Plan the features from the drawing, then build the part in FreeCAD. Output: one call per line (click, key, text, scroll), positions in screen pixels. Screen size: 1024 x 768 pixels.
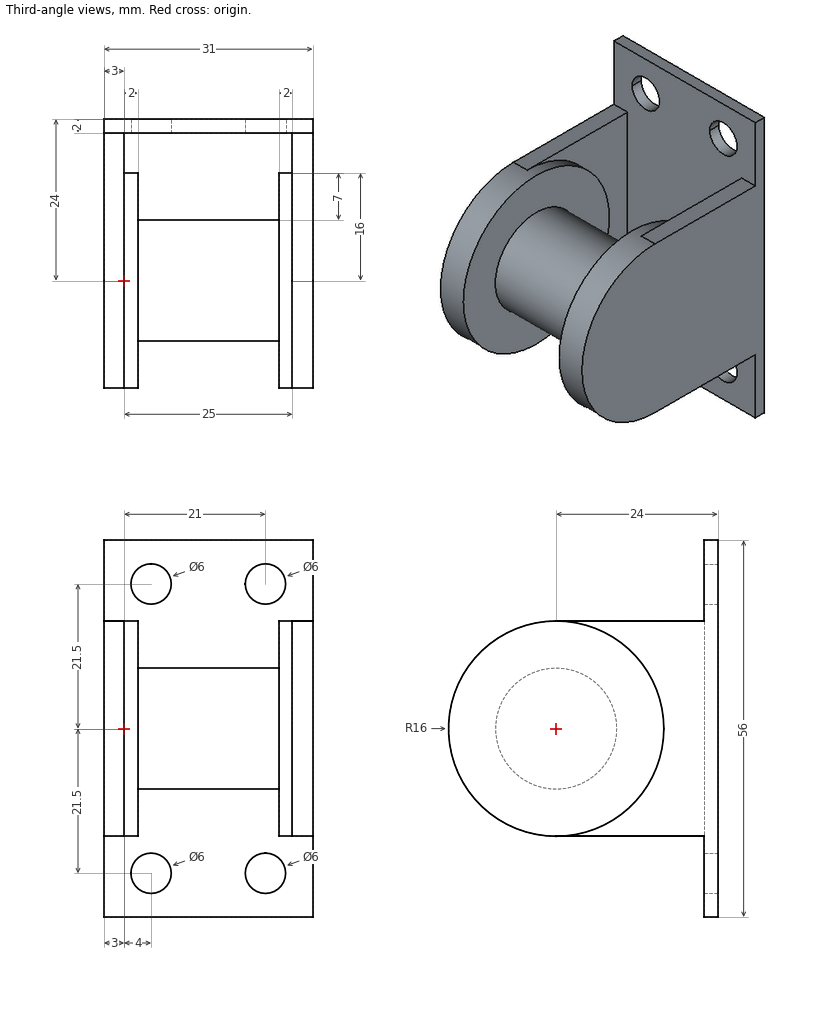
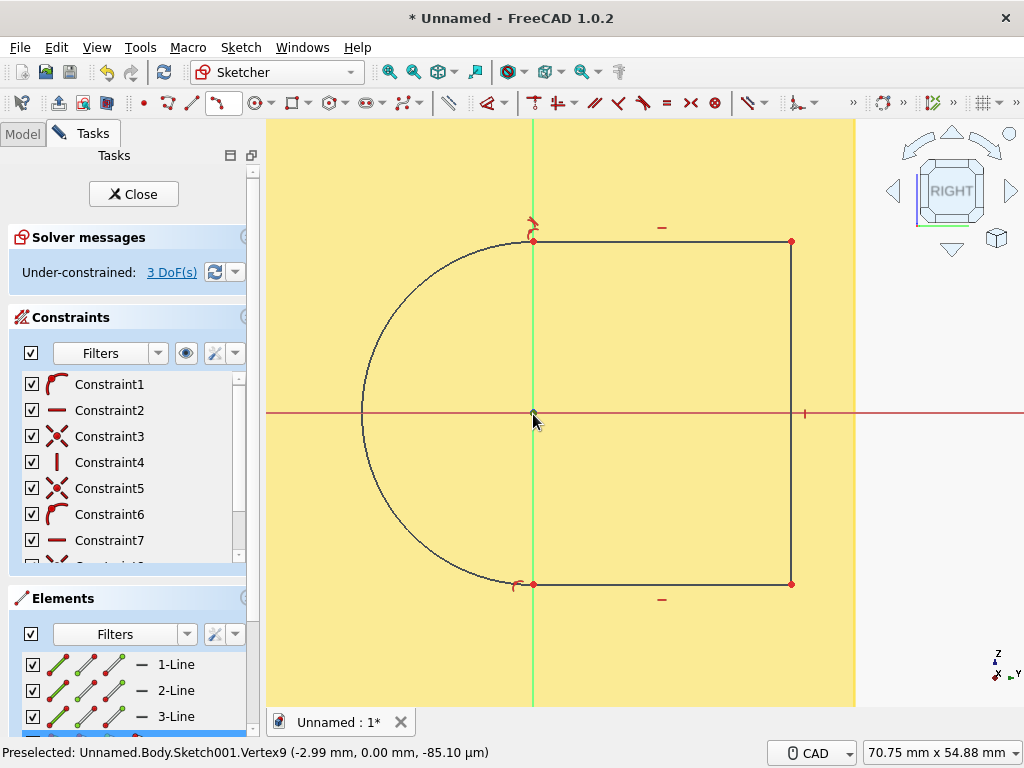
click(415, 413)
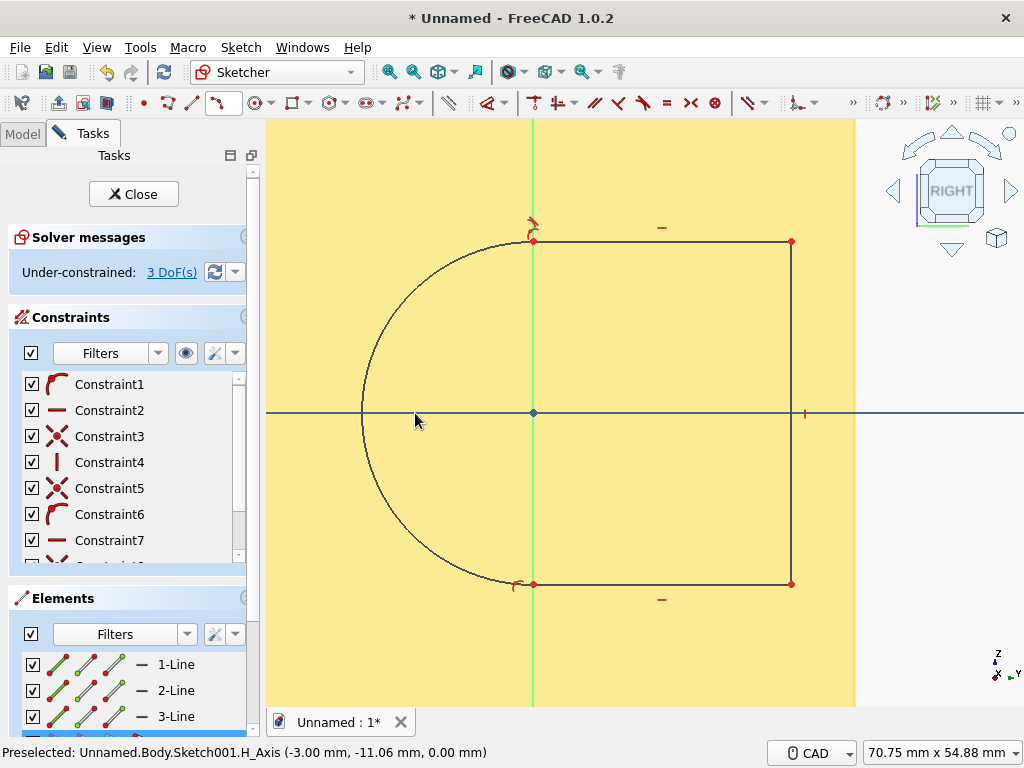
click(534, 104)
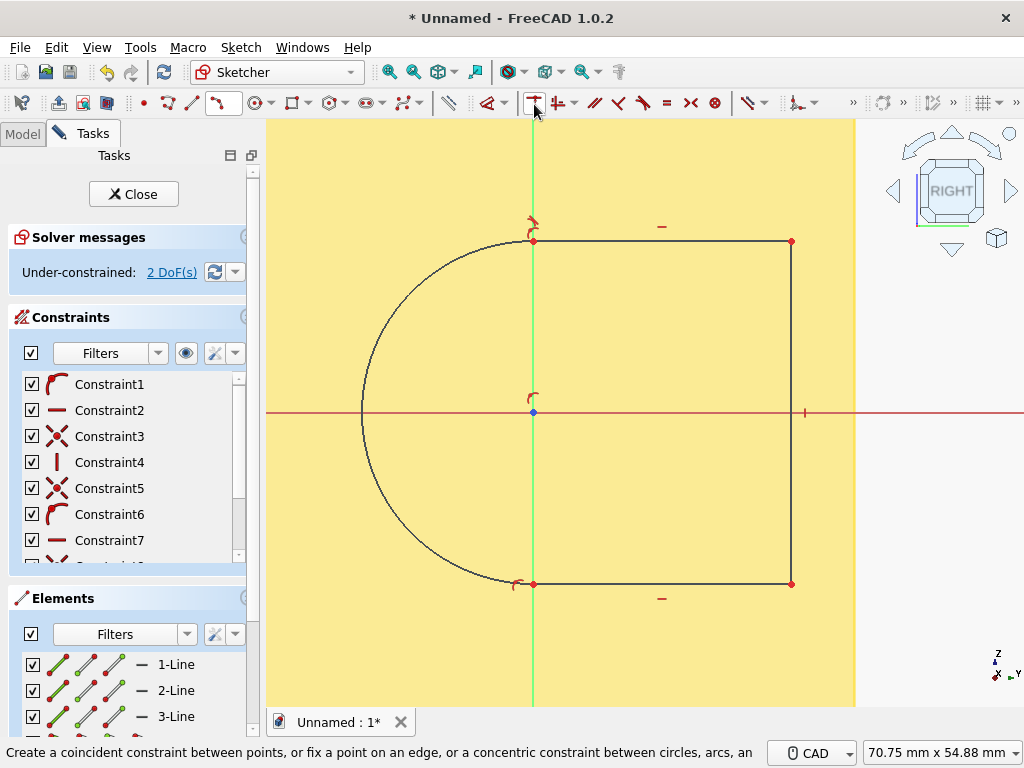
click(488, 104)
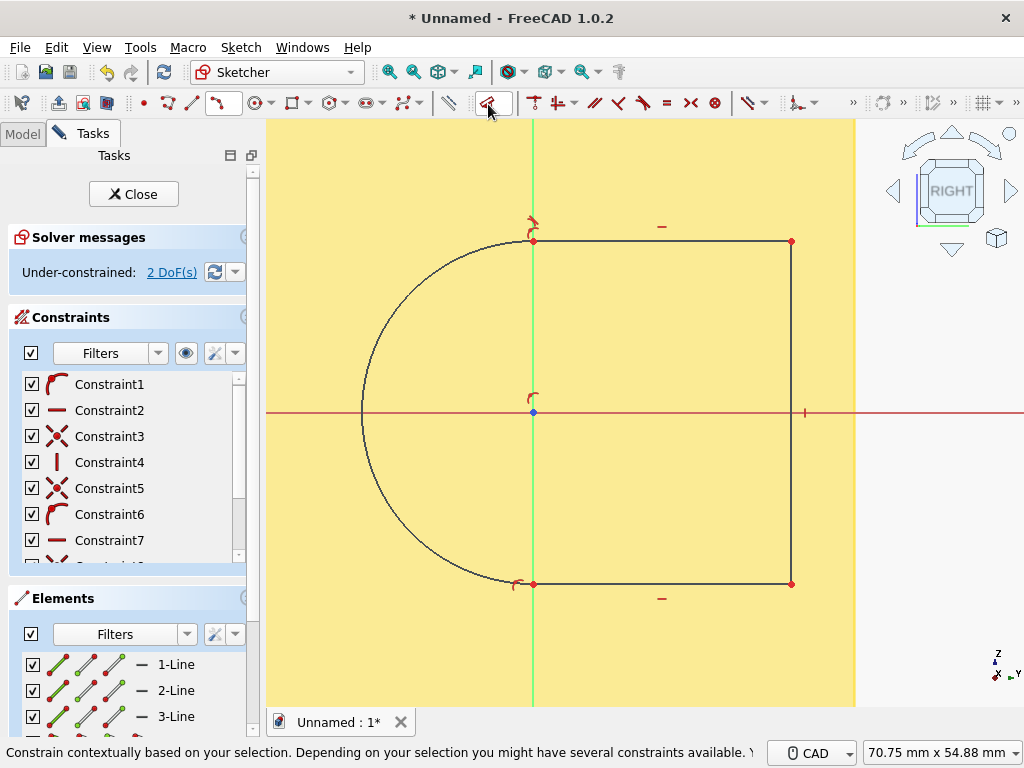
click(395, 312)
click(369, 293)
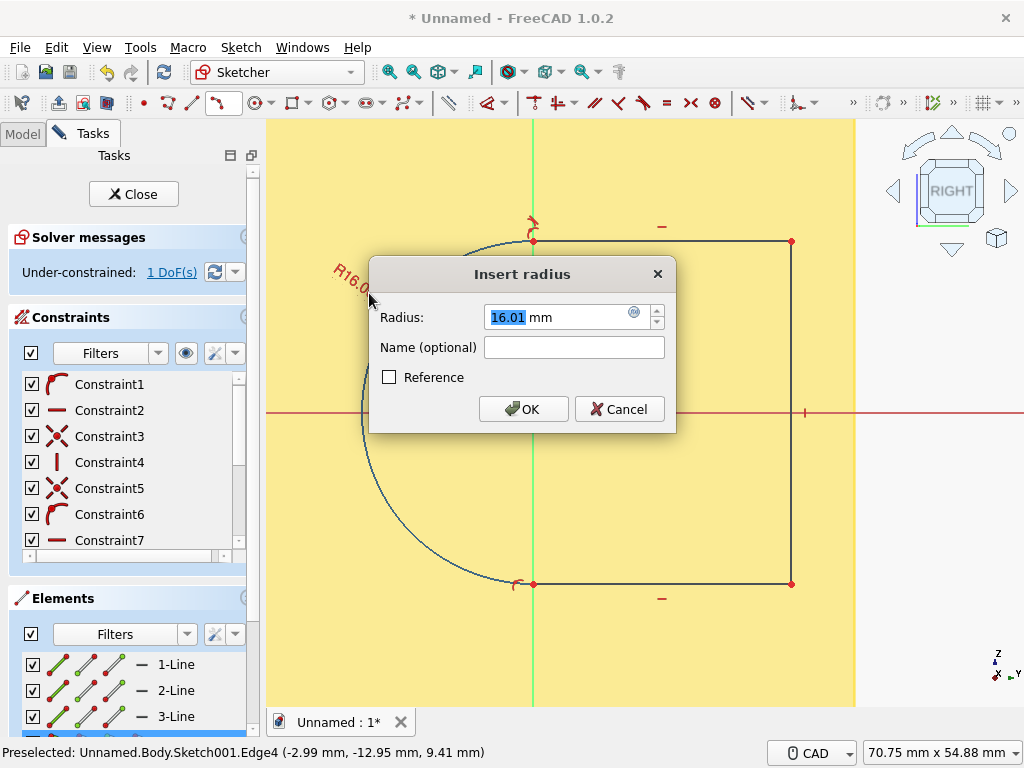
text(16)
key(Return)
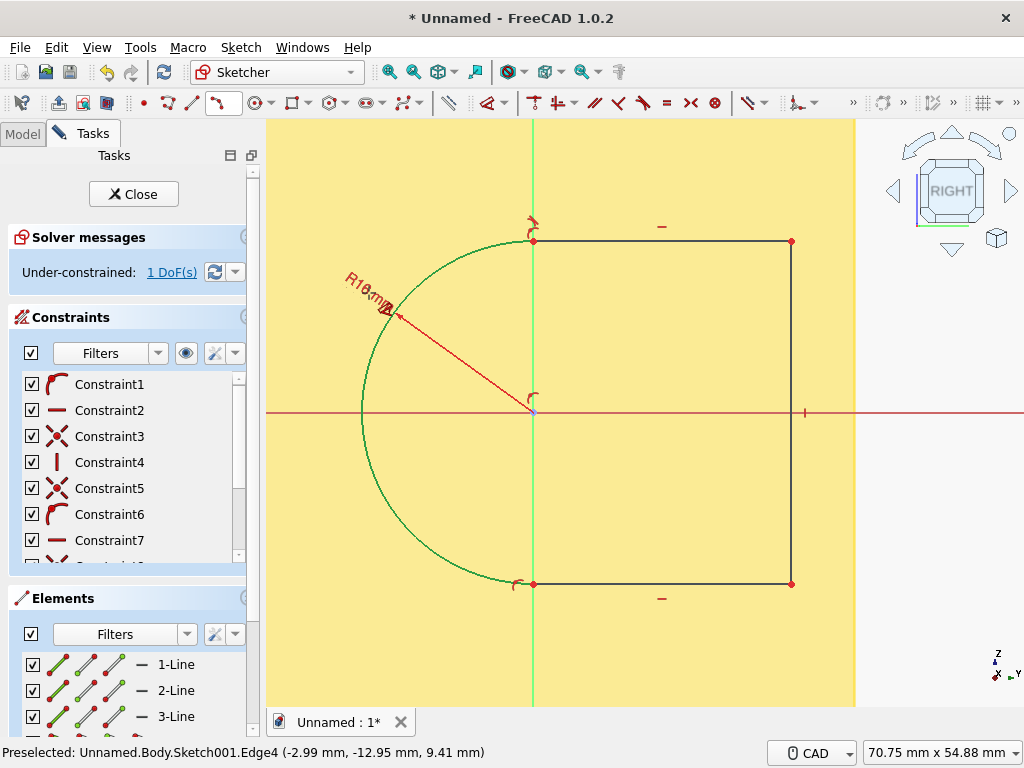
click(611, 241)
click(662, 207)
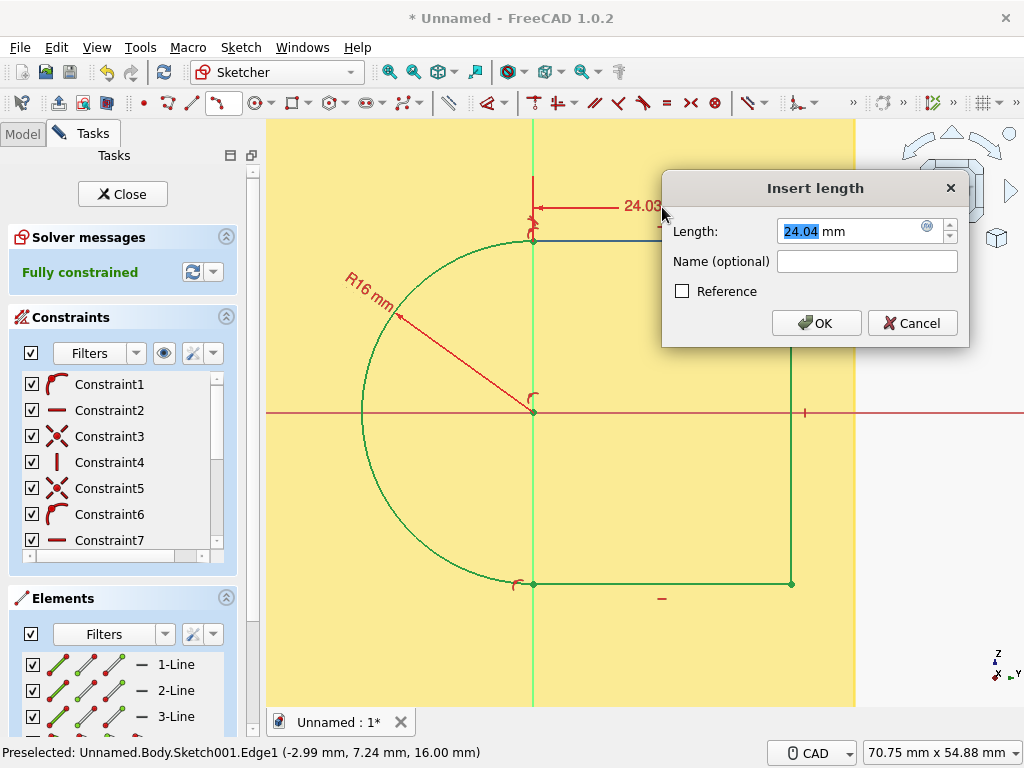
text(24)
key(Return)
key(Escape)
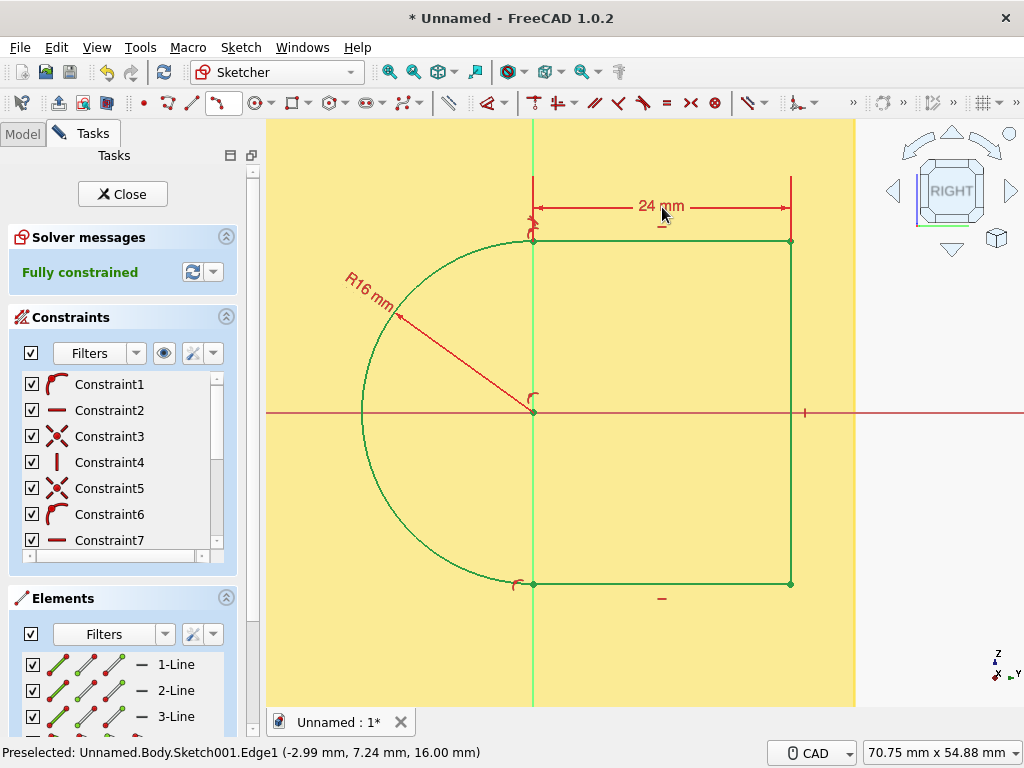
click(123, 194)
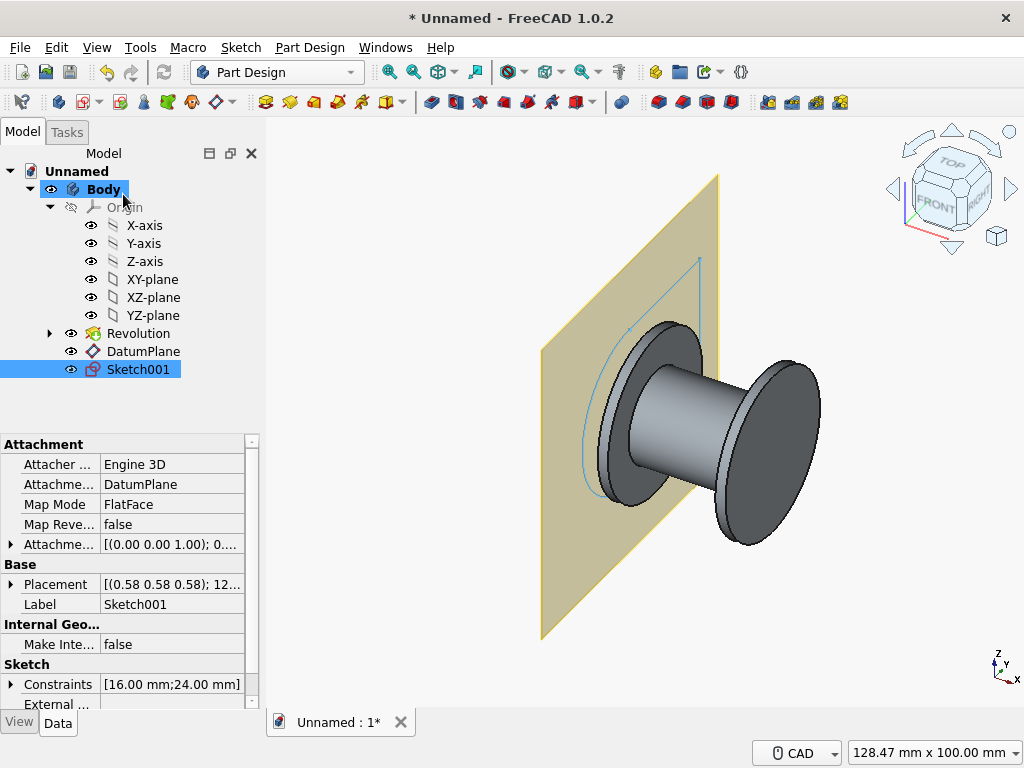
click(266, 102)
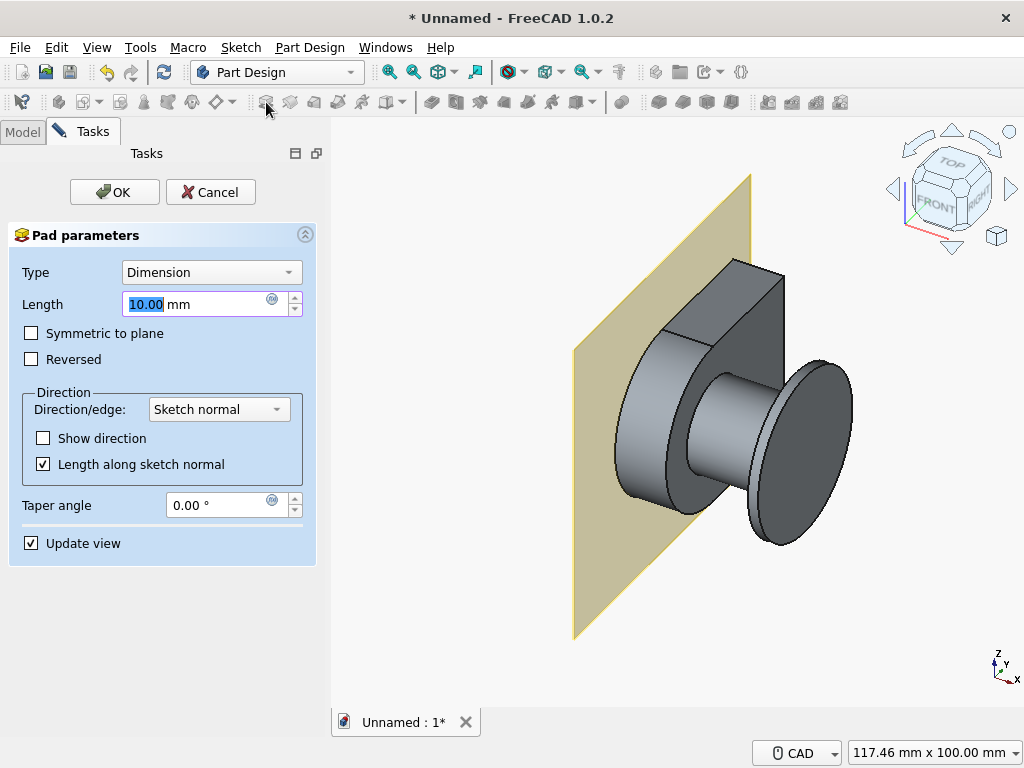
text(3)
key(Tab)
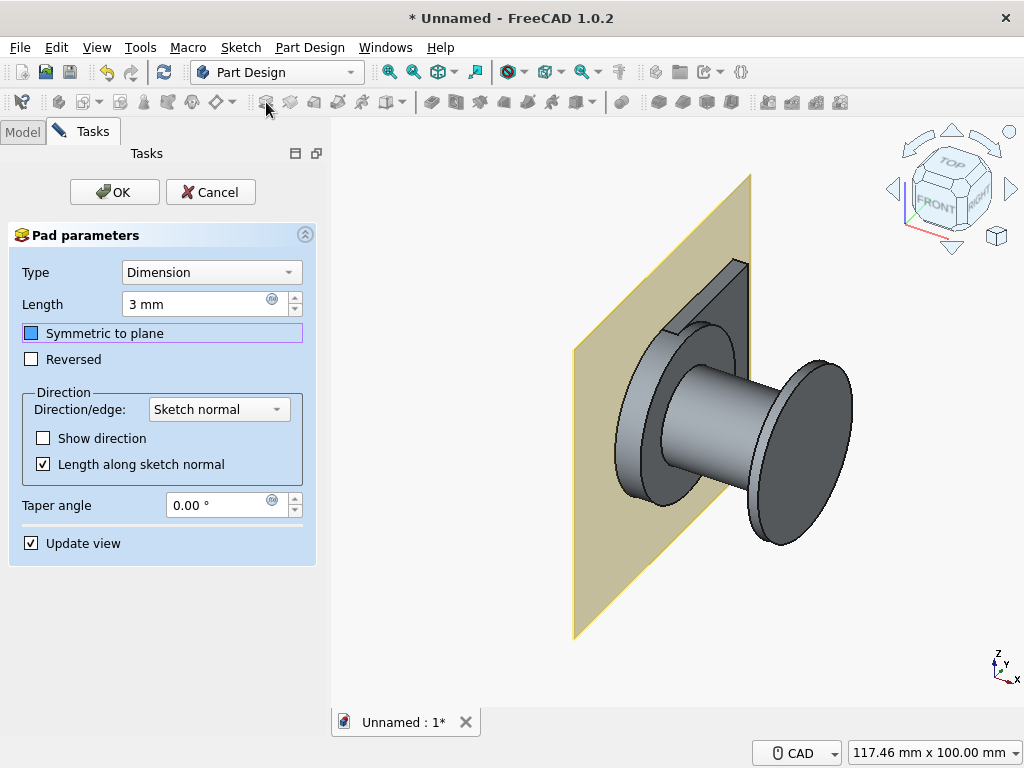
click(115, 192)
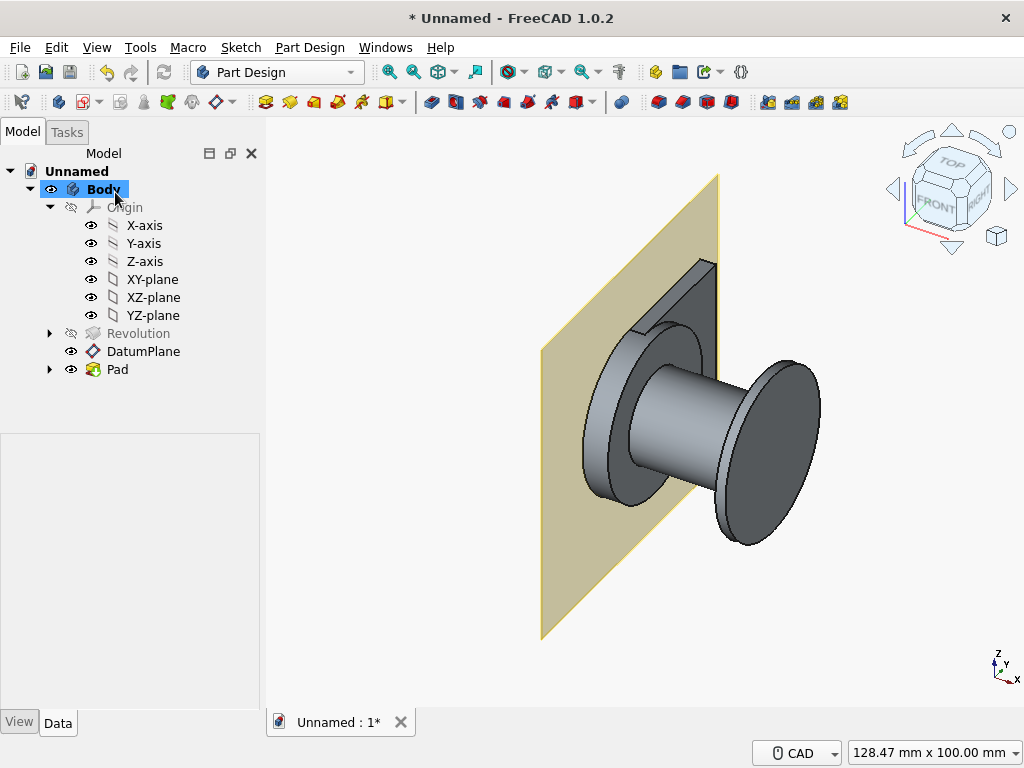
click(116, 351)
key(space)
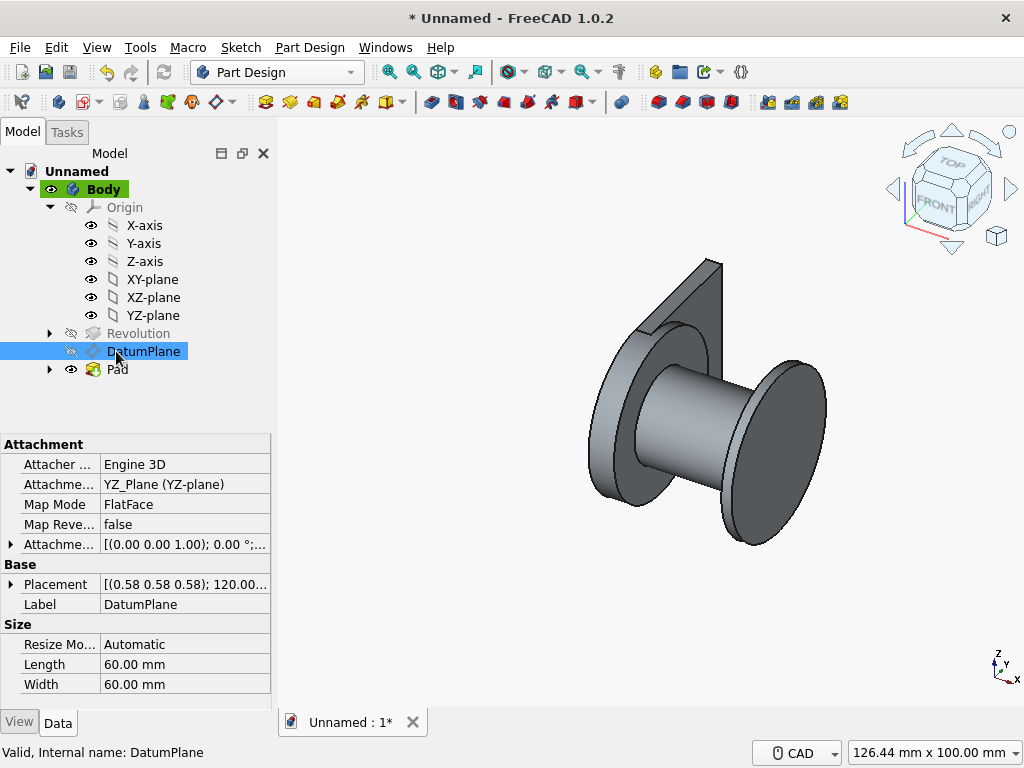
click(136, 315)